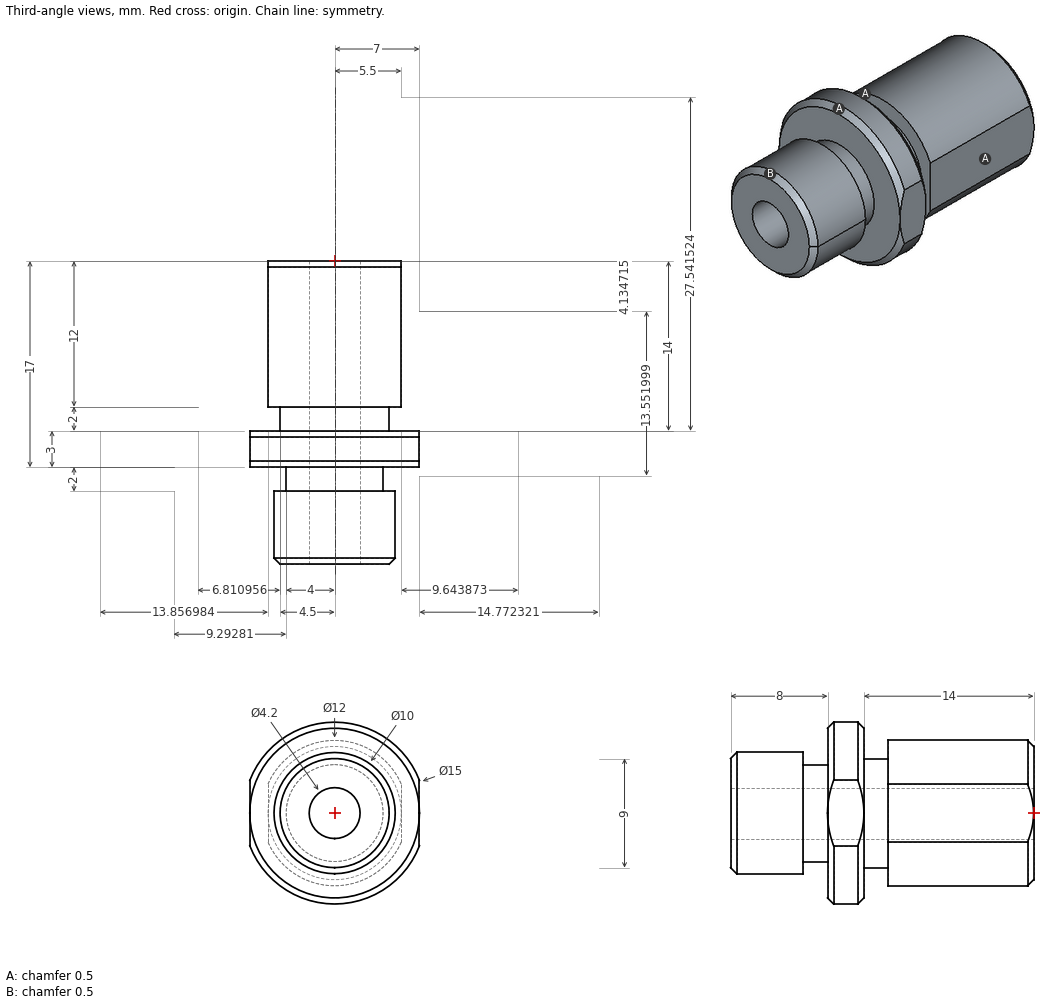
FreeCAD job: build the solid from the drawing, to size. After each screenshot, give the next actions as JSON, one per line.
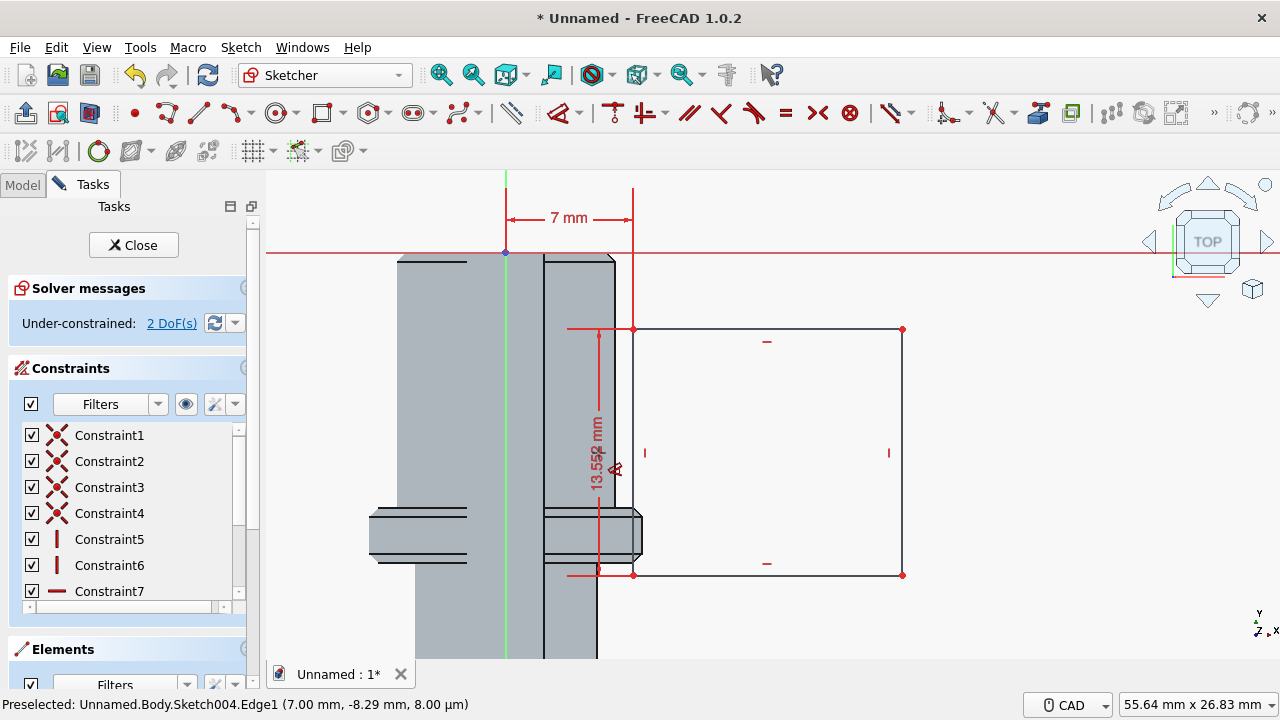
{"action": "left_click", "coordinate": [714, 576]}
{"action": "left_click", "coordinate": [768, 610]}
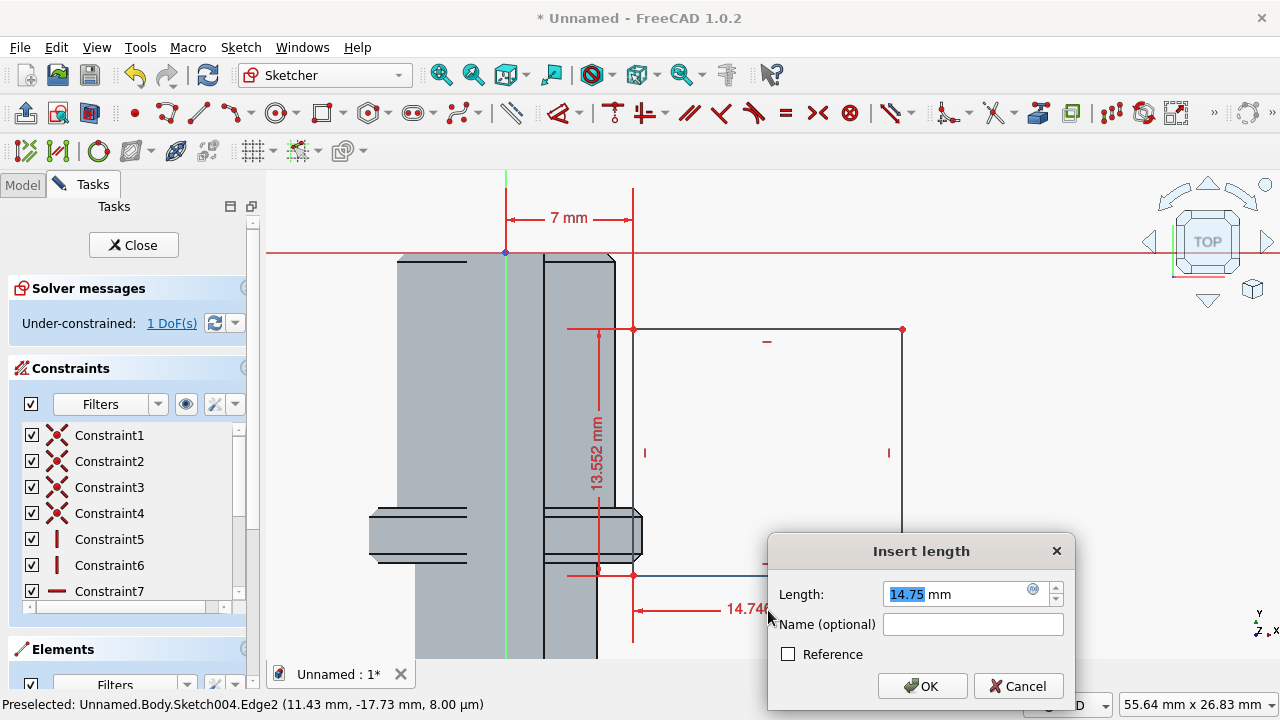
{"action": "type", "text": "14.772321"}
{"action": "key", "text": "Return"}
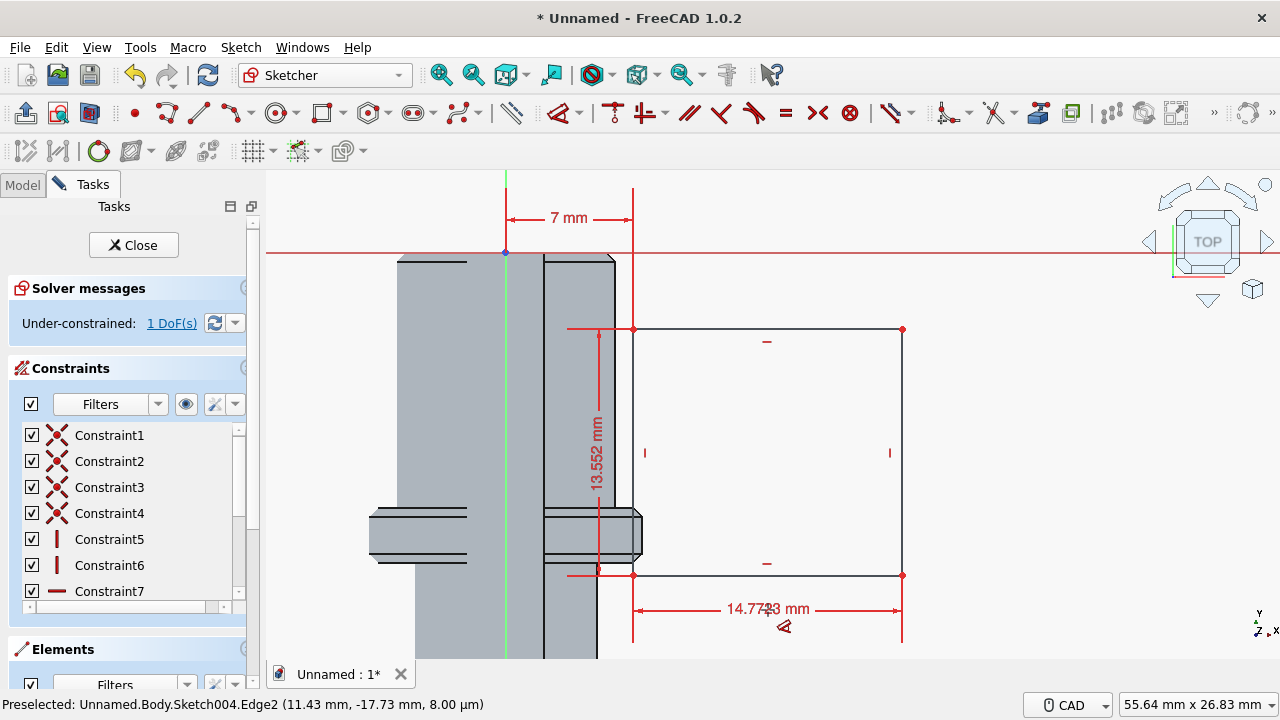
{"action": "left_click", "coordinate": [633, 329]}
{"action": "left_click", "coordinate": [472, 291]}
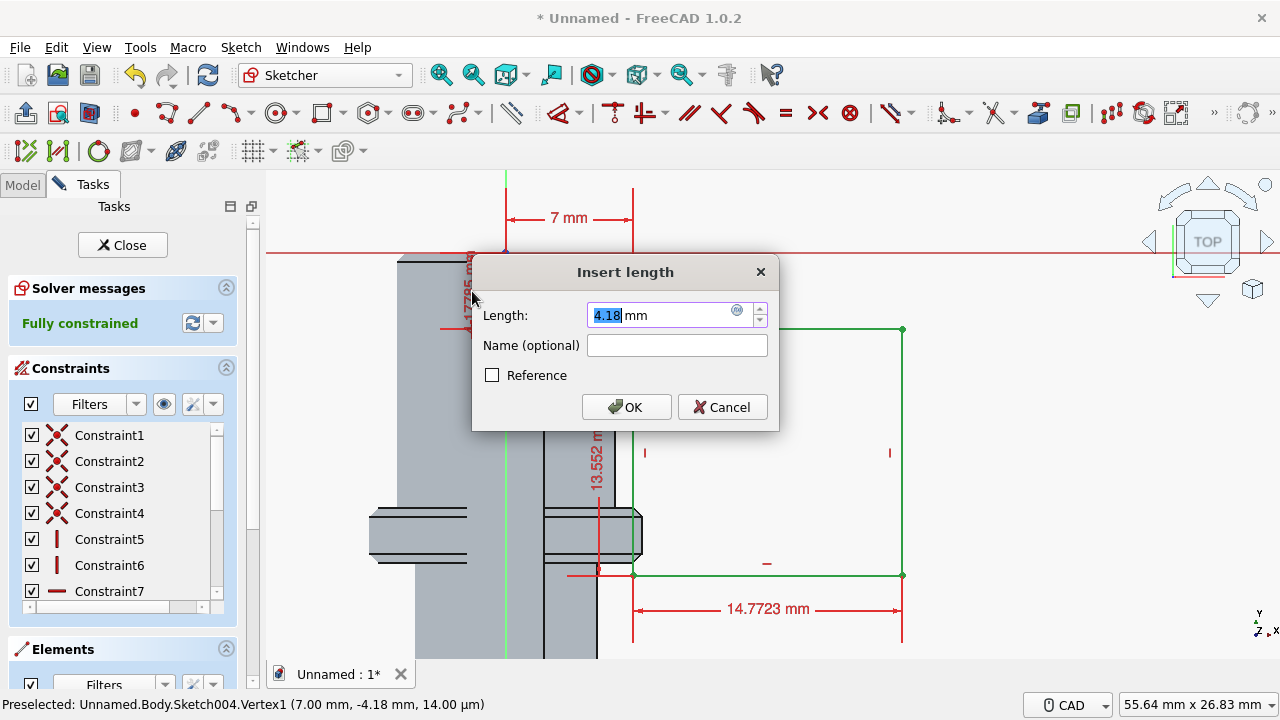
{"action": "type", "text": "4.134715"}
{"action": "key", "text": "Return"}
{"action": "key", "text": "Escape"}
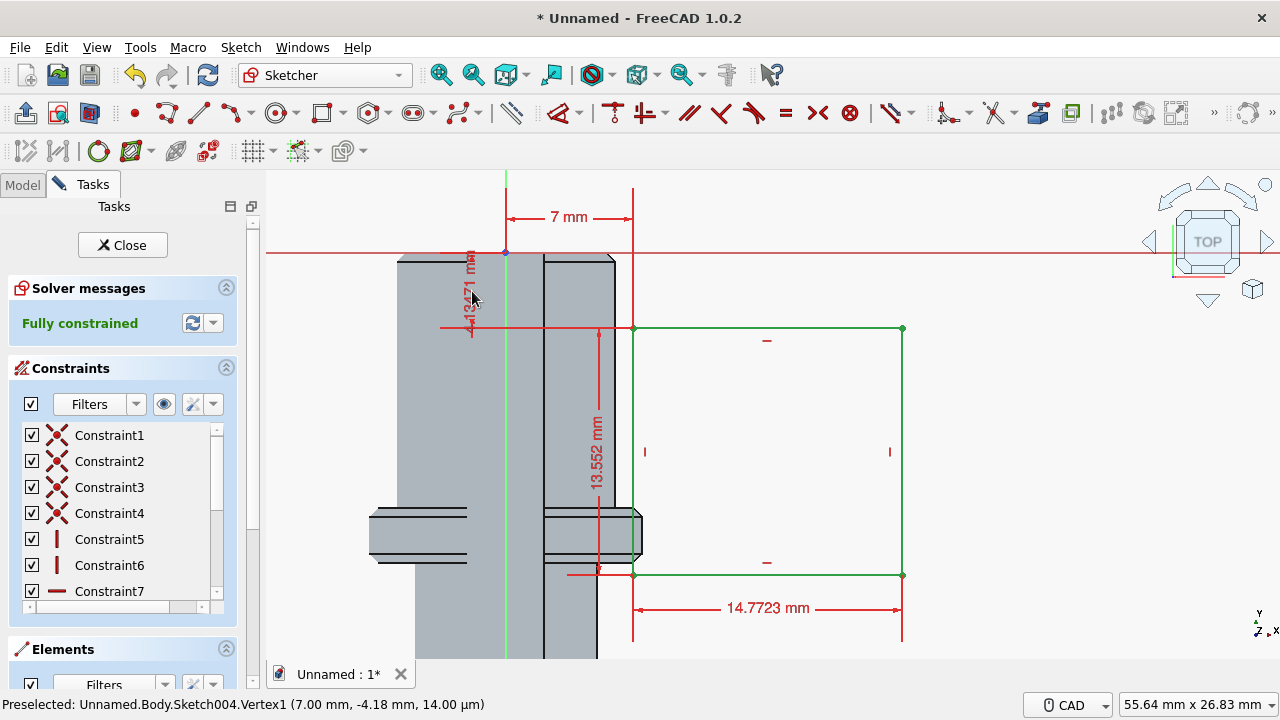
{"action": "left_click", "coordinate": [123, 245]}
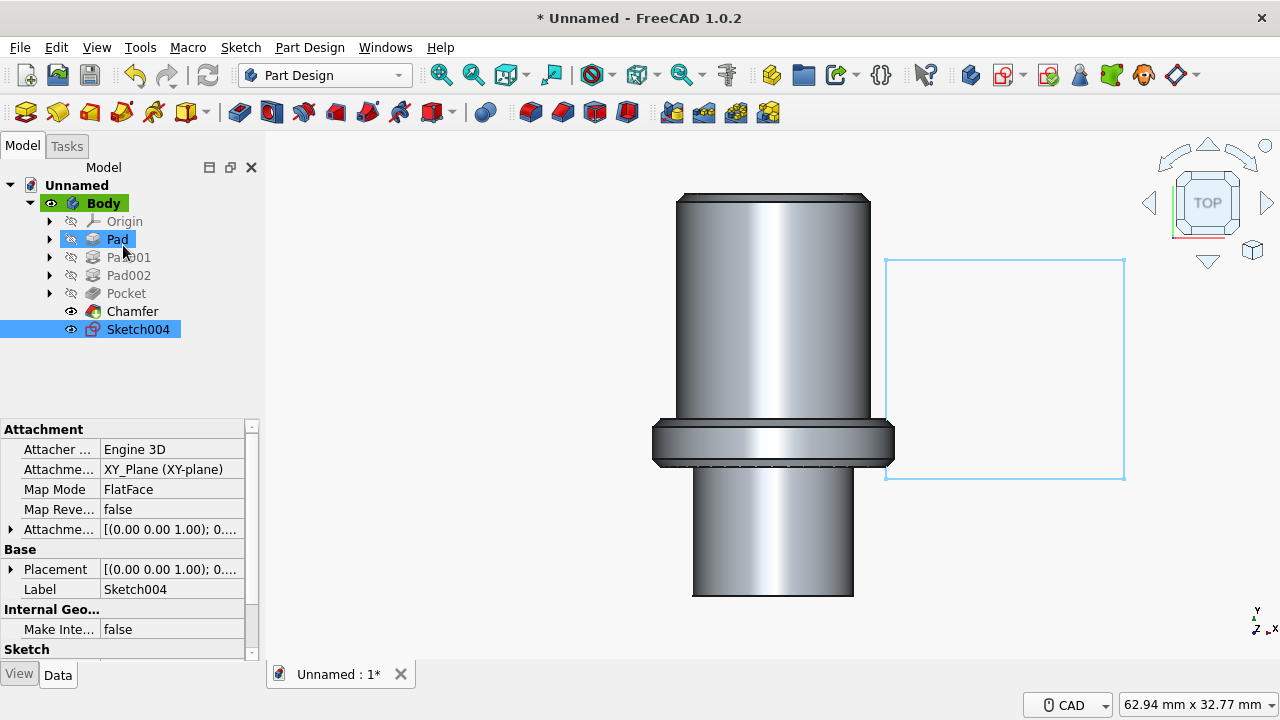
{"action": "left_click", "coordinate": [240, 112]}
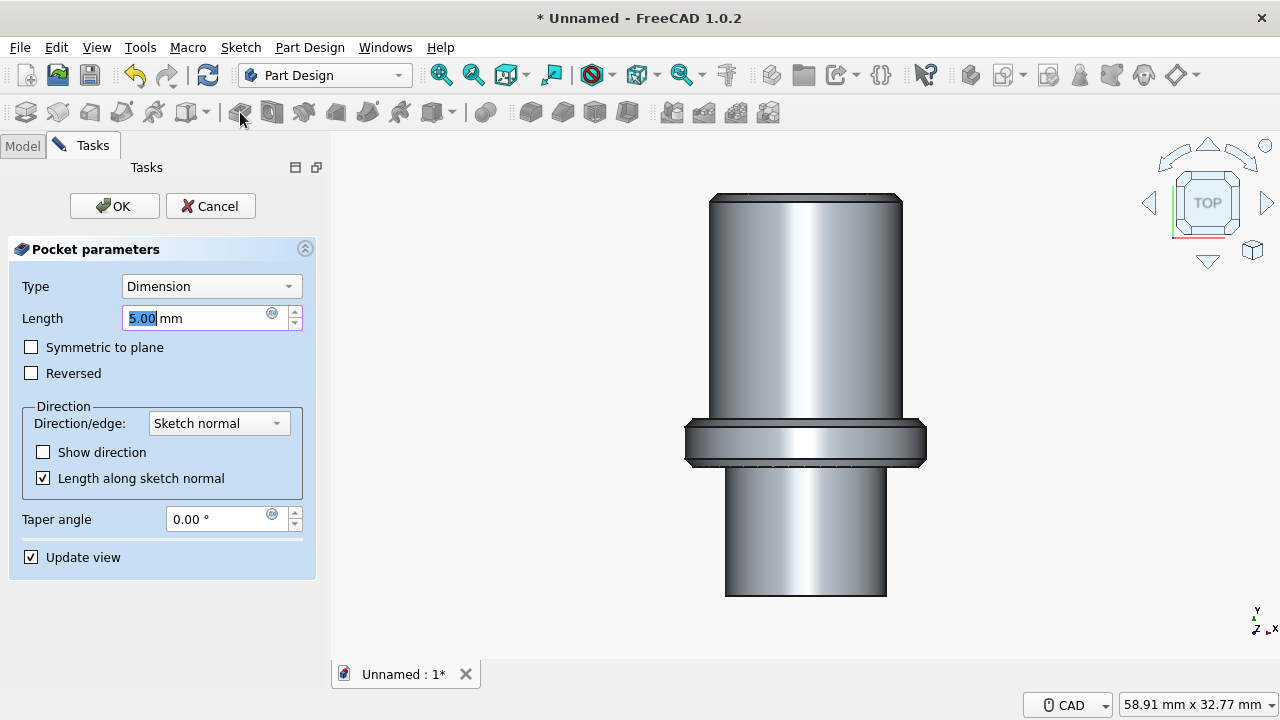
{"action": "type", "text": "9"}
{"action": "key", "text": "Tab"}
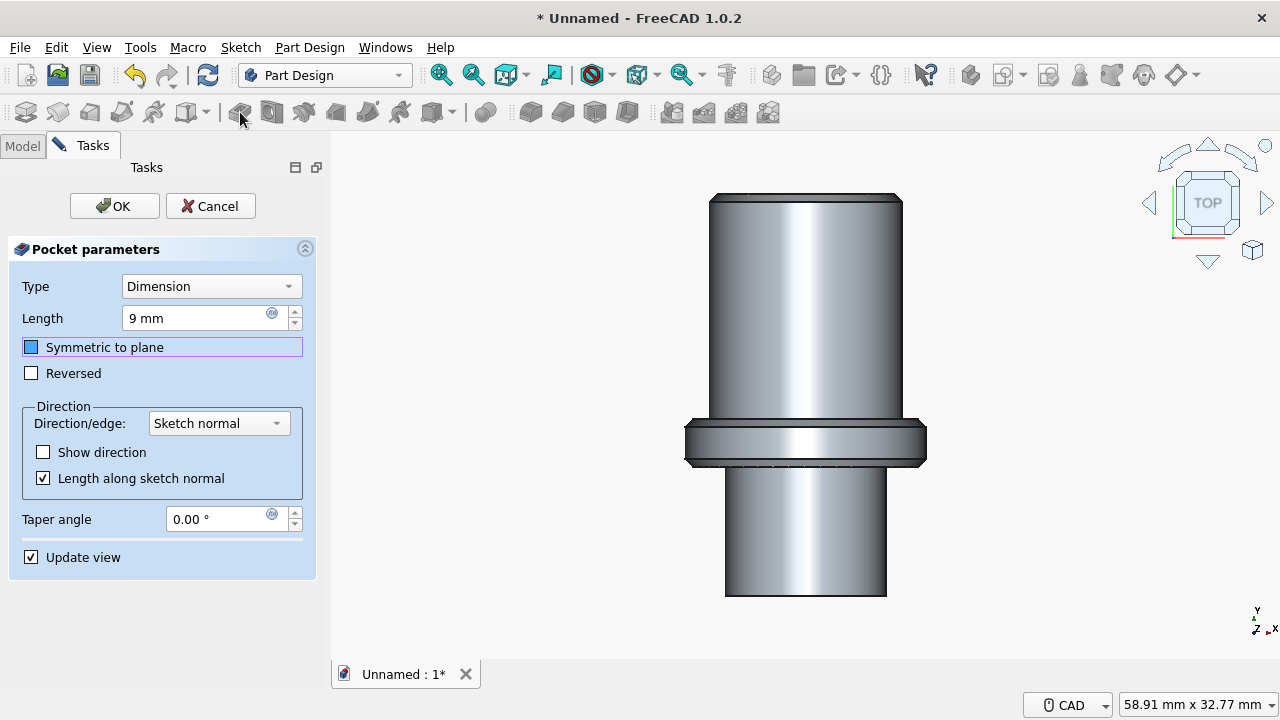
{"action": "left_click", "coordinate": [30, 347]}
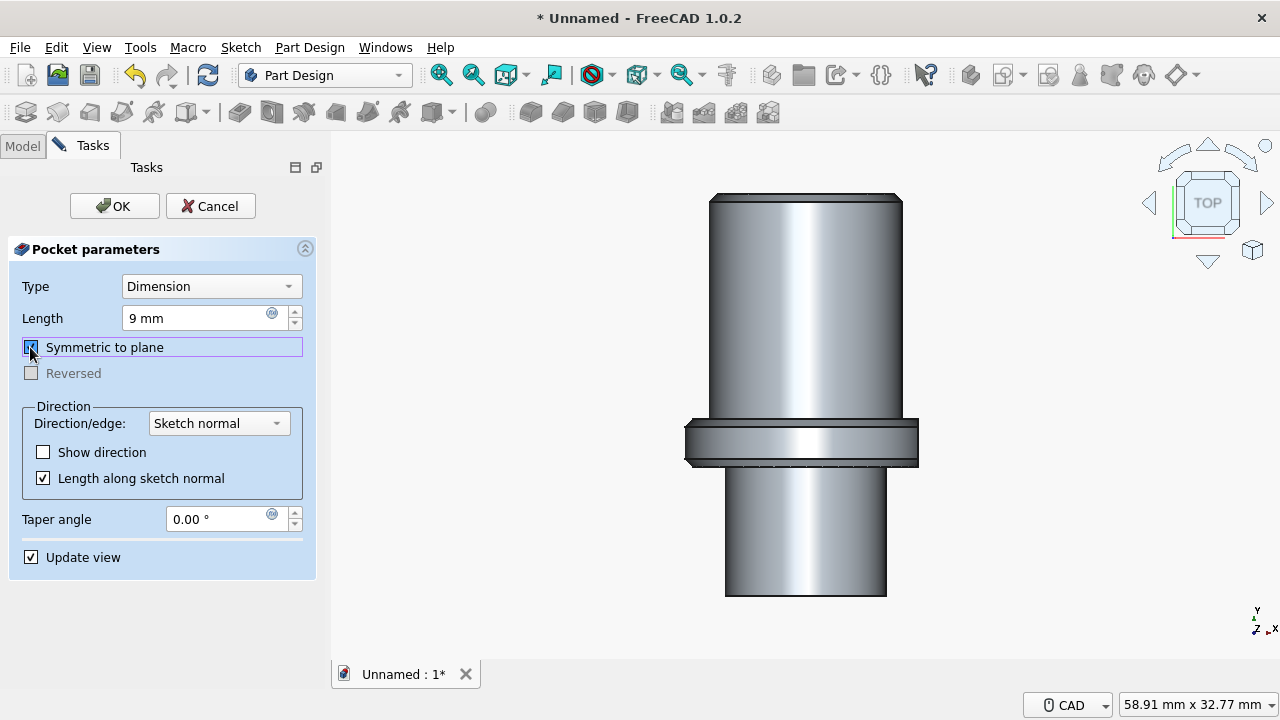
{"action": "left_click", "coordinate": [115, 206]}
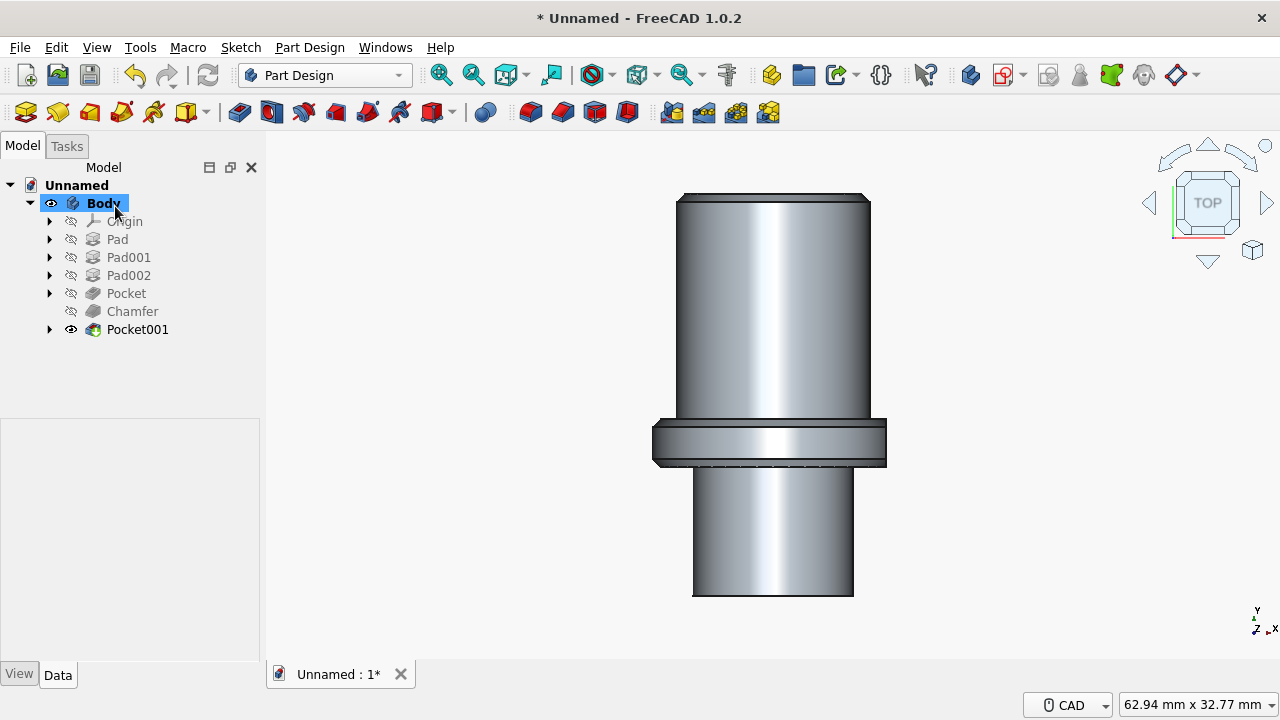
{"action": "left_click", "coordinate": [116, 329]}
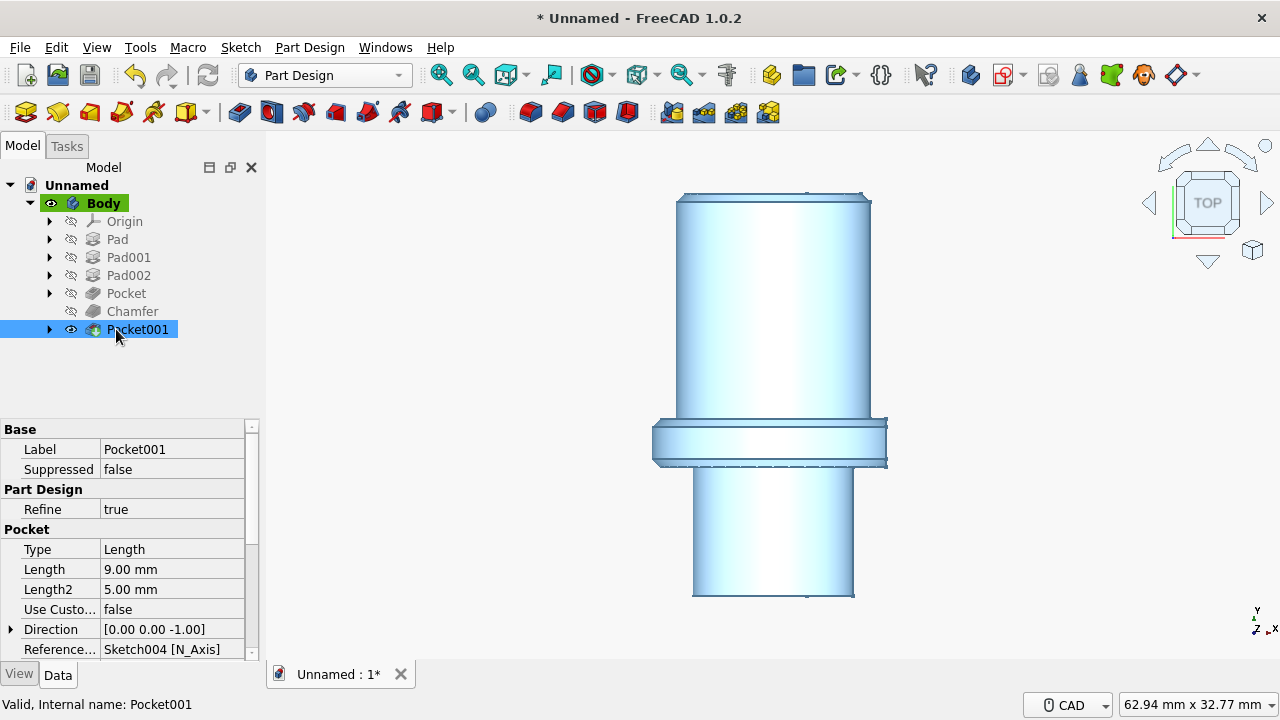
{"action": "left_click", "coordinate": [672, 112]}